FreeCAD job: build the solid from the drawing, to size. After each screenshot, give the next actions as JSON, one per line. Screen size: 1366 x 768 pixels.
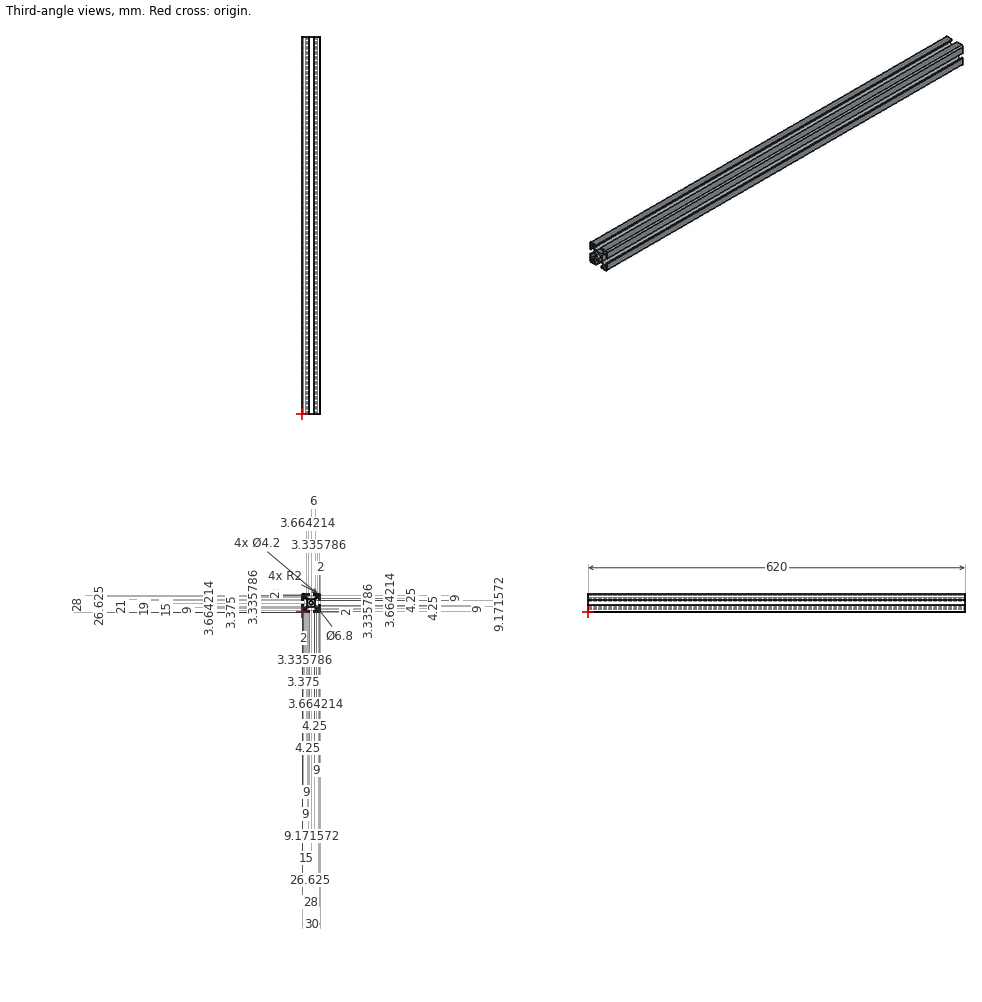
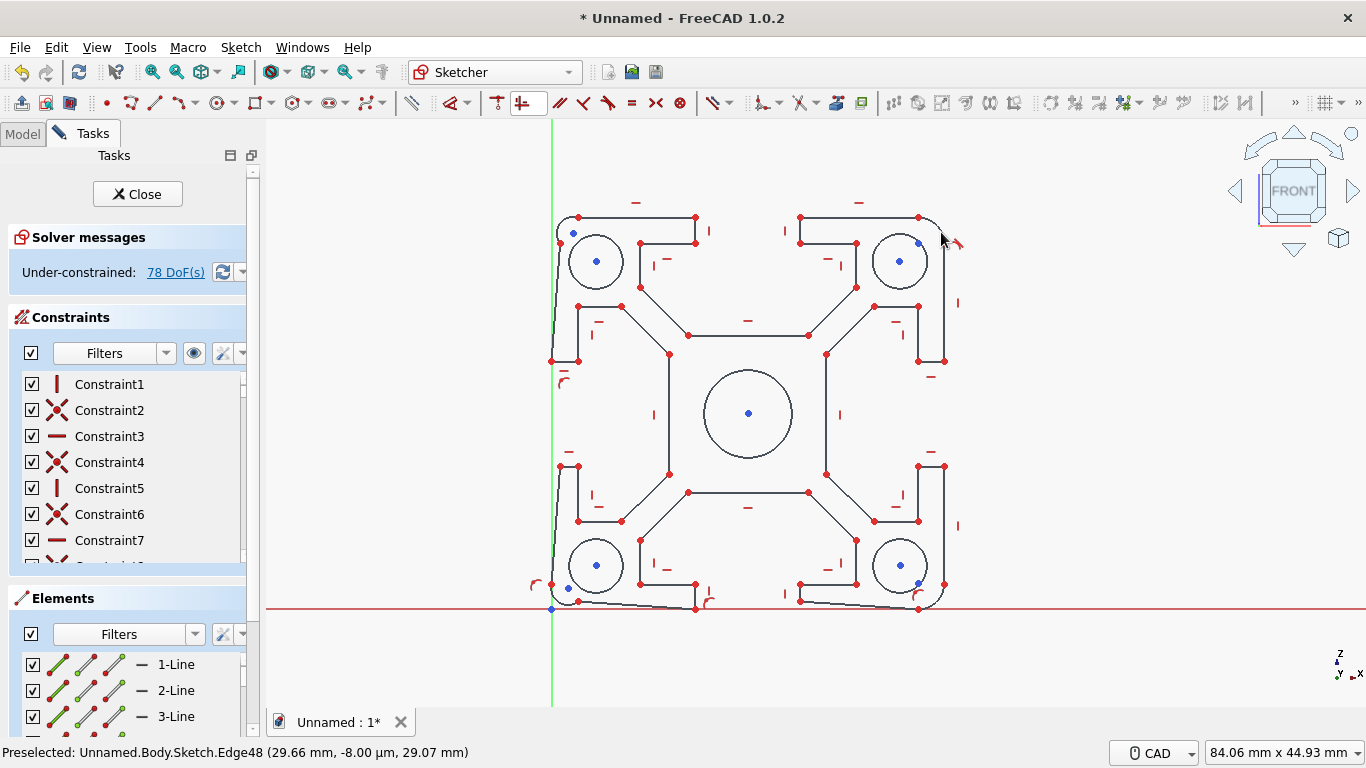
{"action": "left_click", "coordinate": [944, 502]}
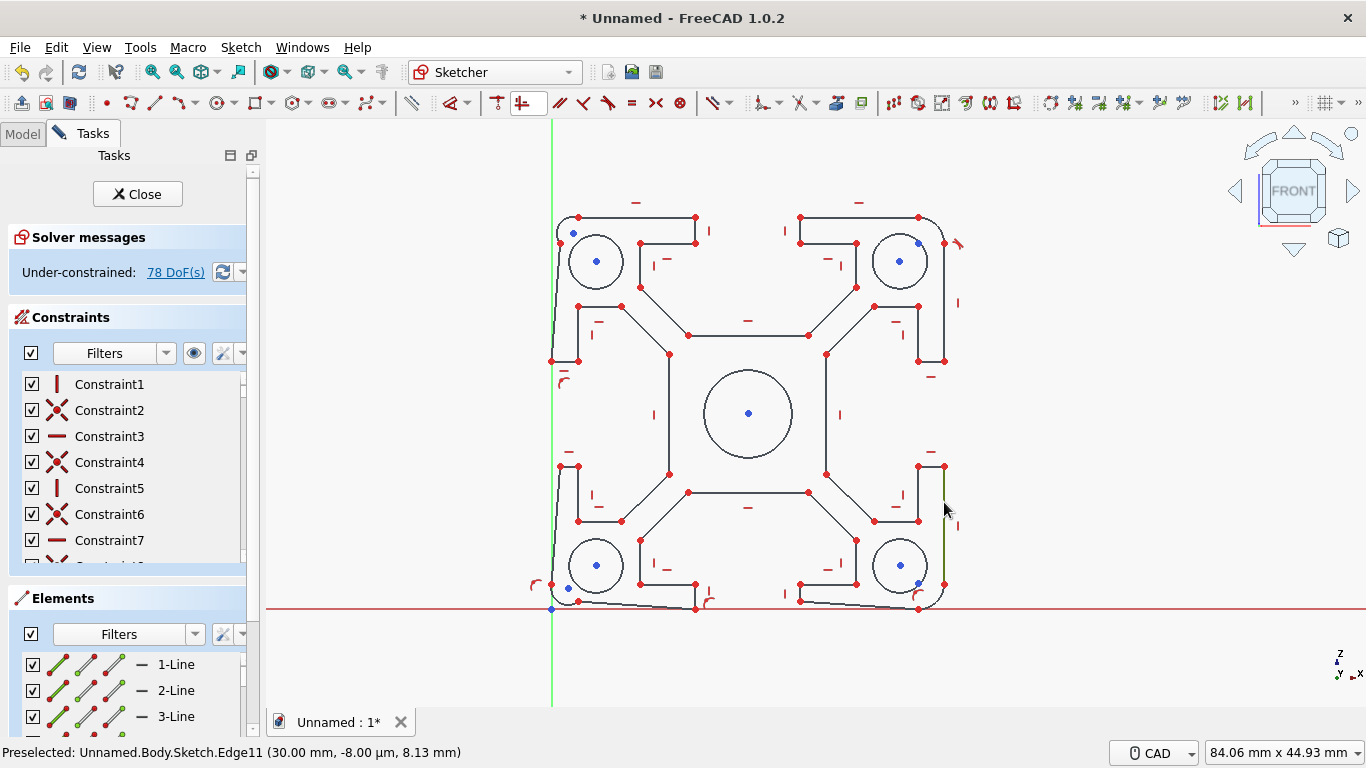
{"action": "left_click", "coordinate": [930, 607]}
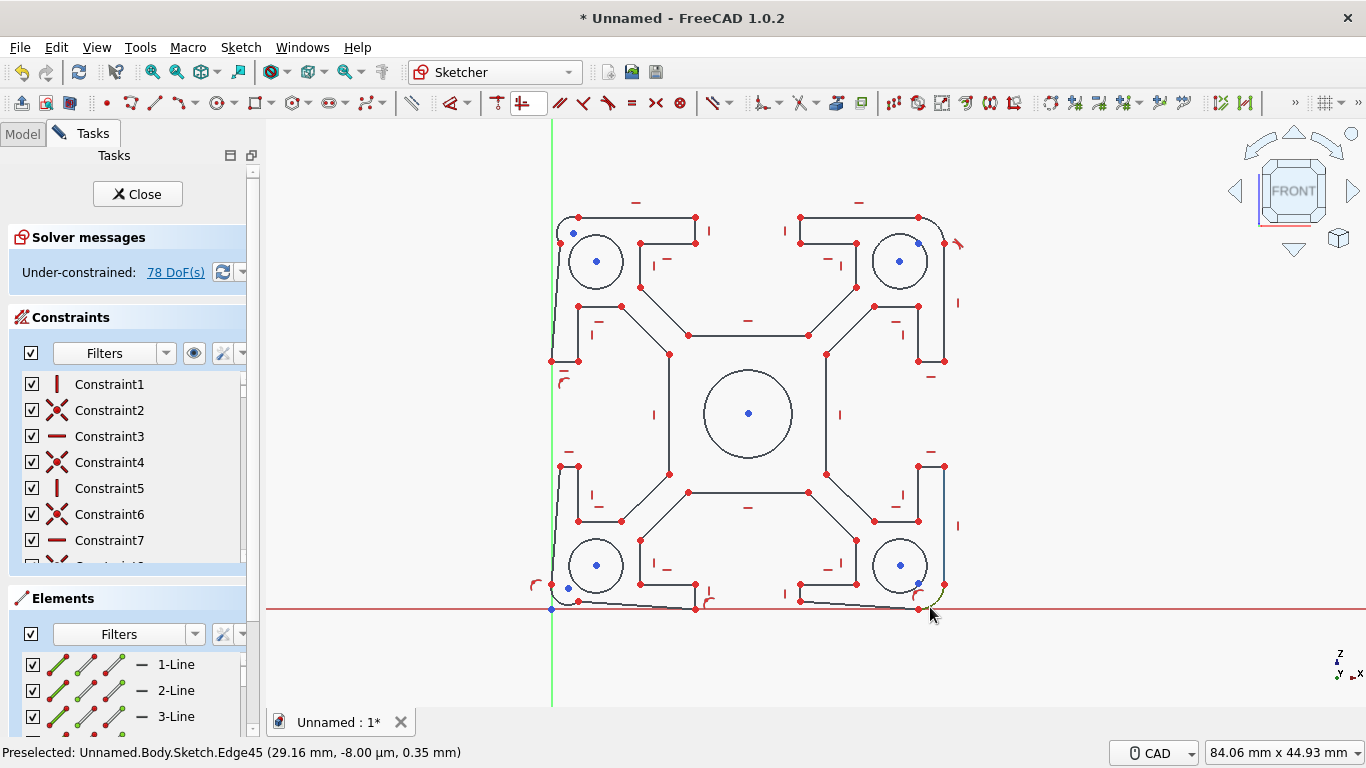
{"action": "key", "text": "t"}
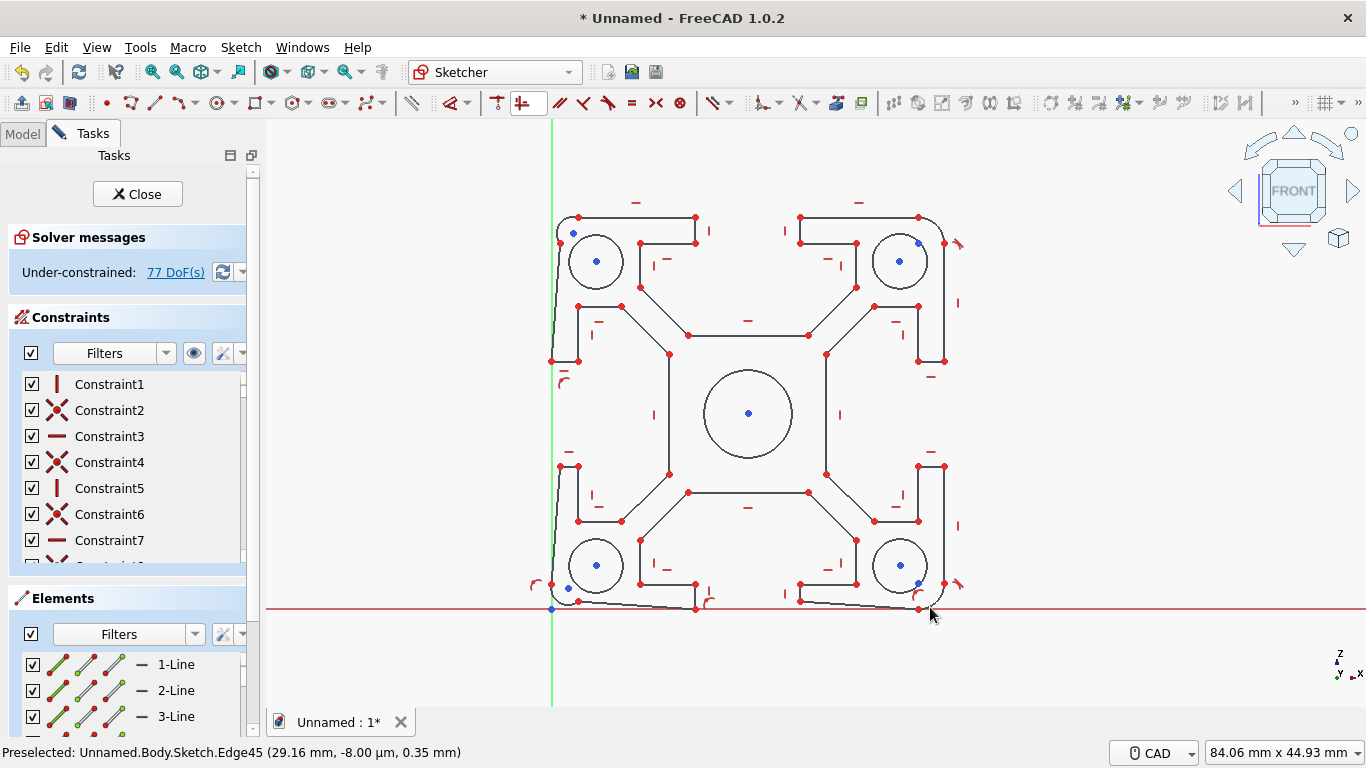
{"action": "left_click", "coordinate": [883, 607]}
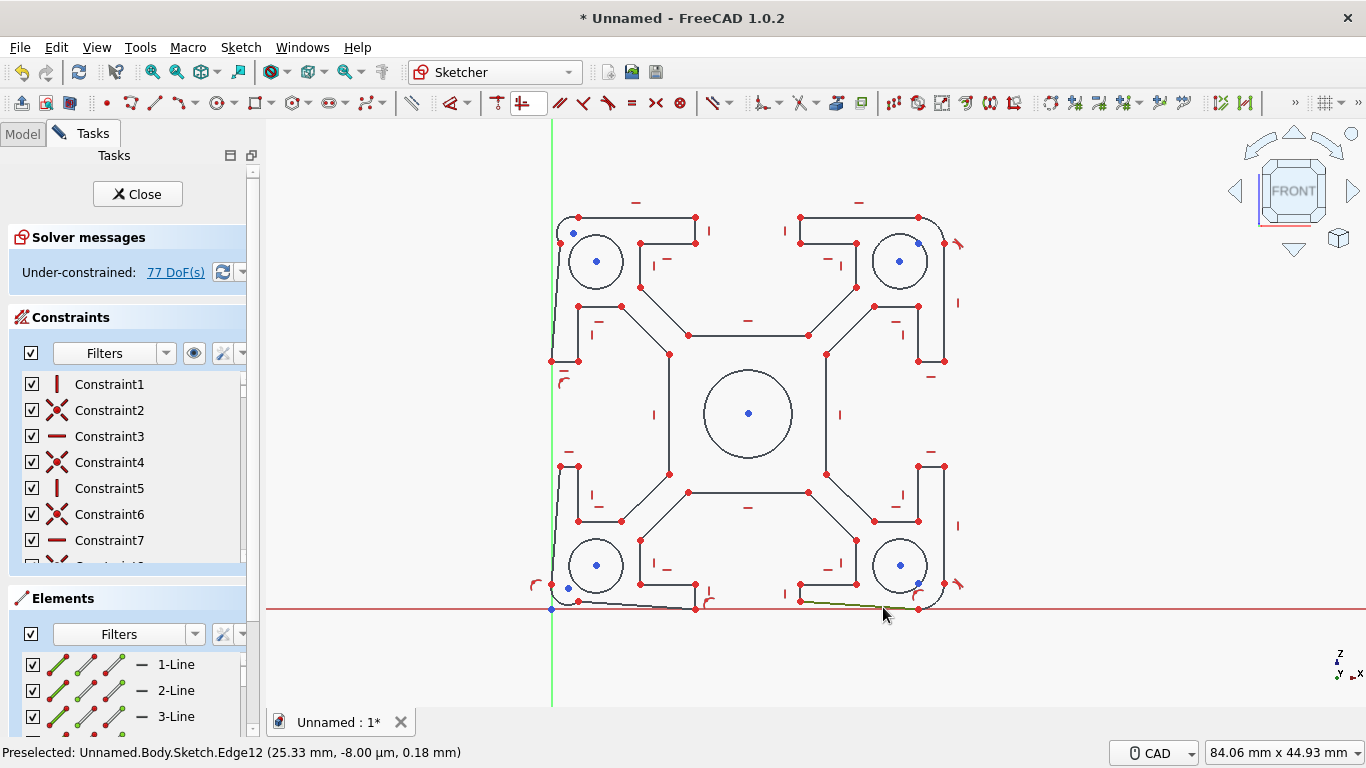
{"action": "left_click", "coordinate": [930, 607]}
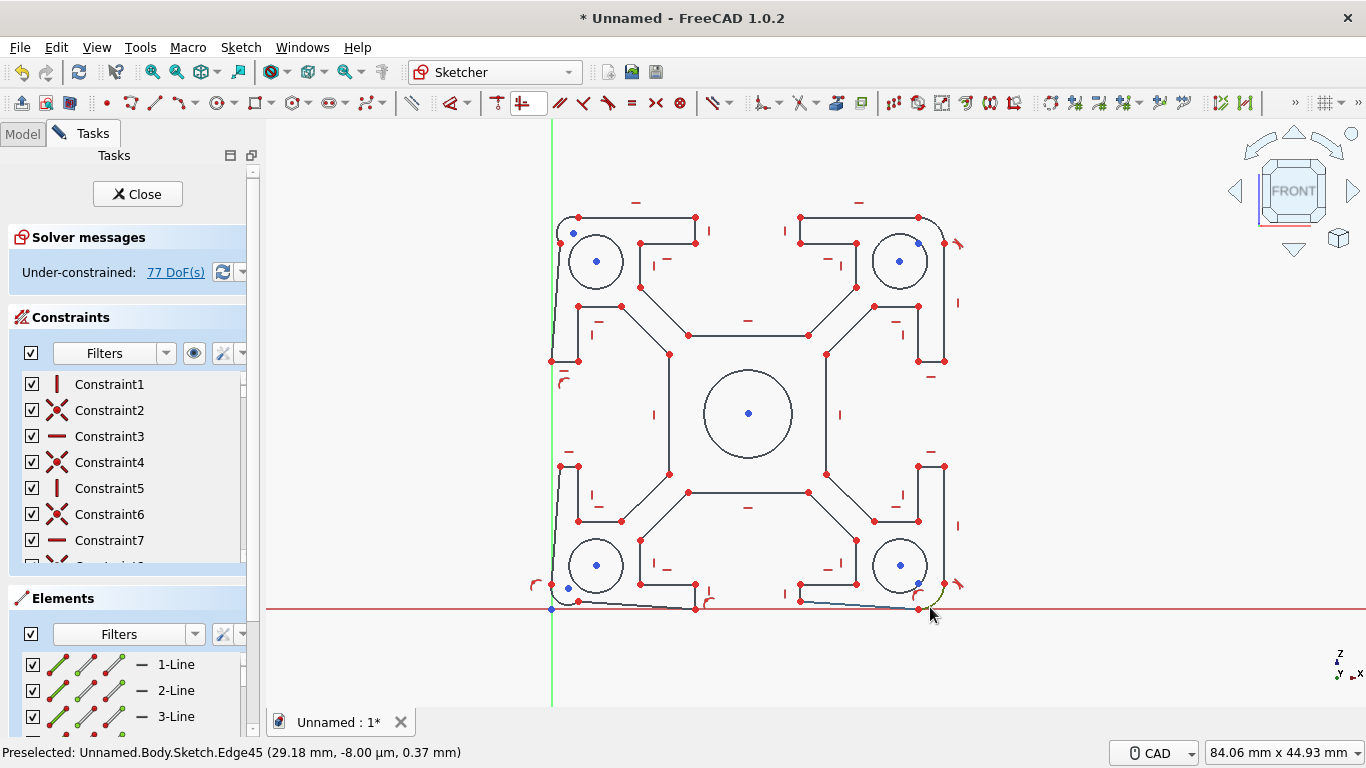
{"action": "key", "text": "t"}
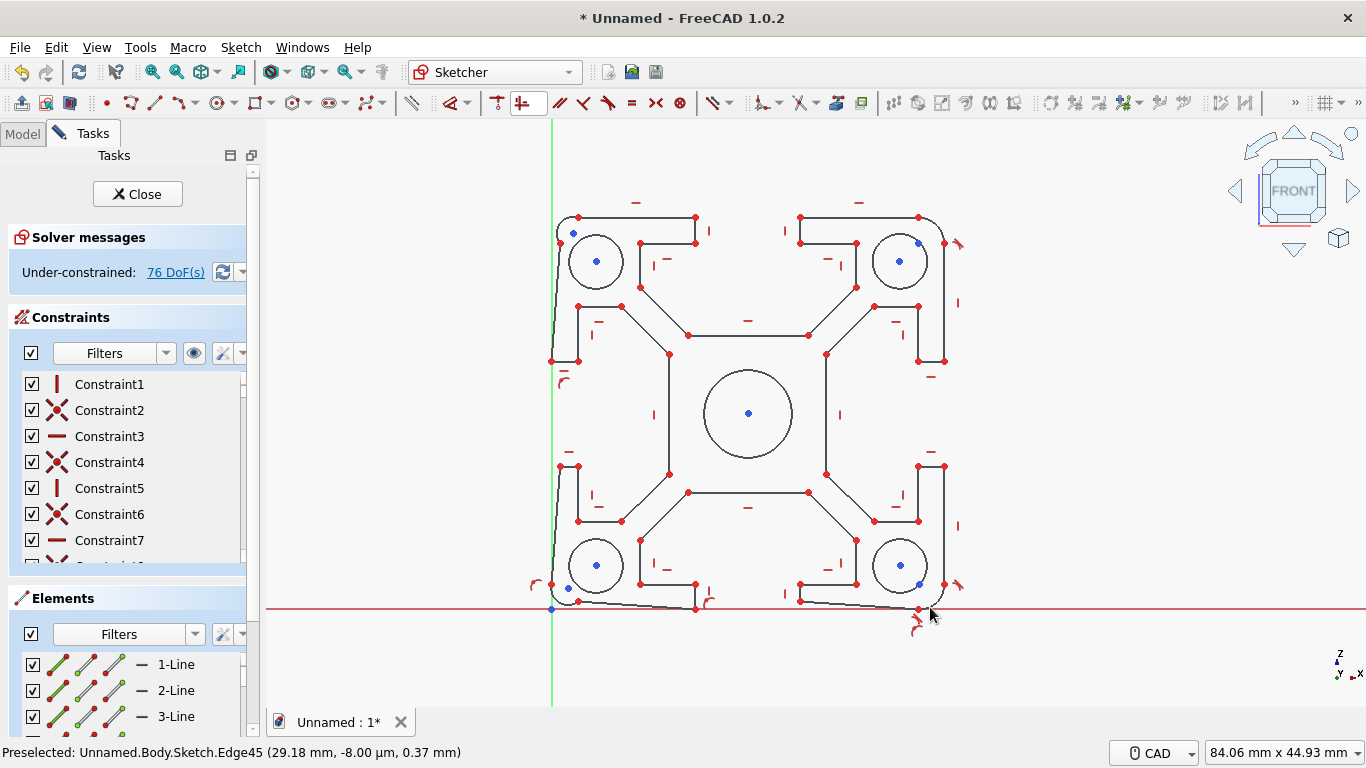
{"action": "left_click", "coordinate": [660, 607]}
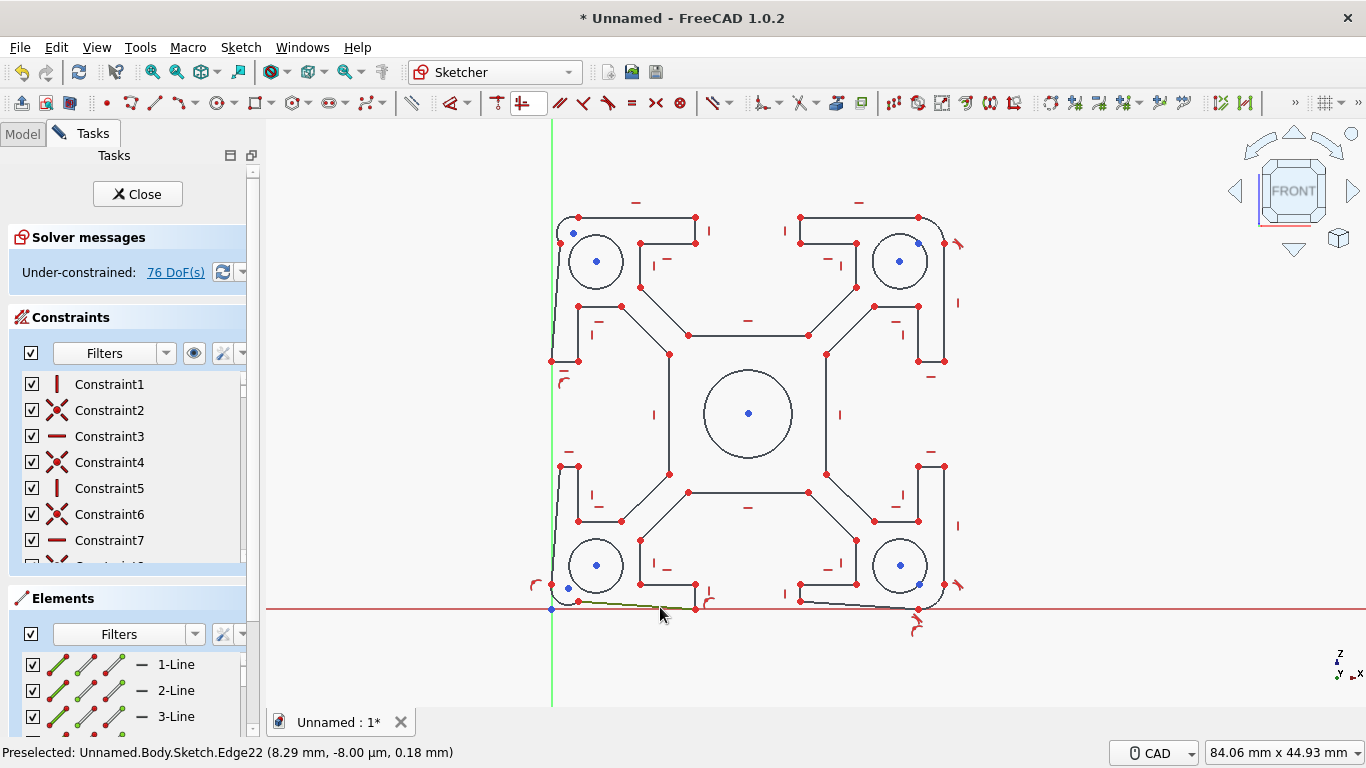
{"action": "left_click", "coordinate": [553, 596]}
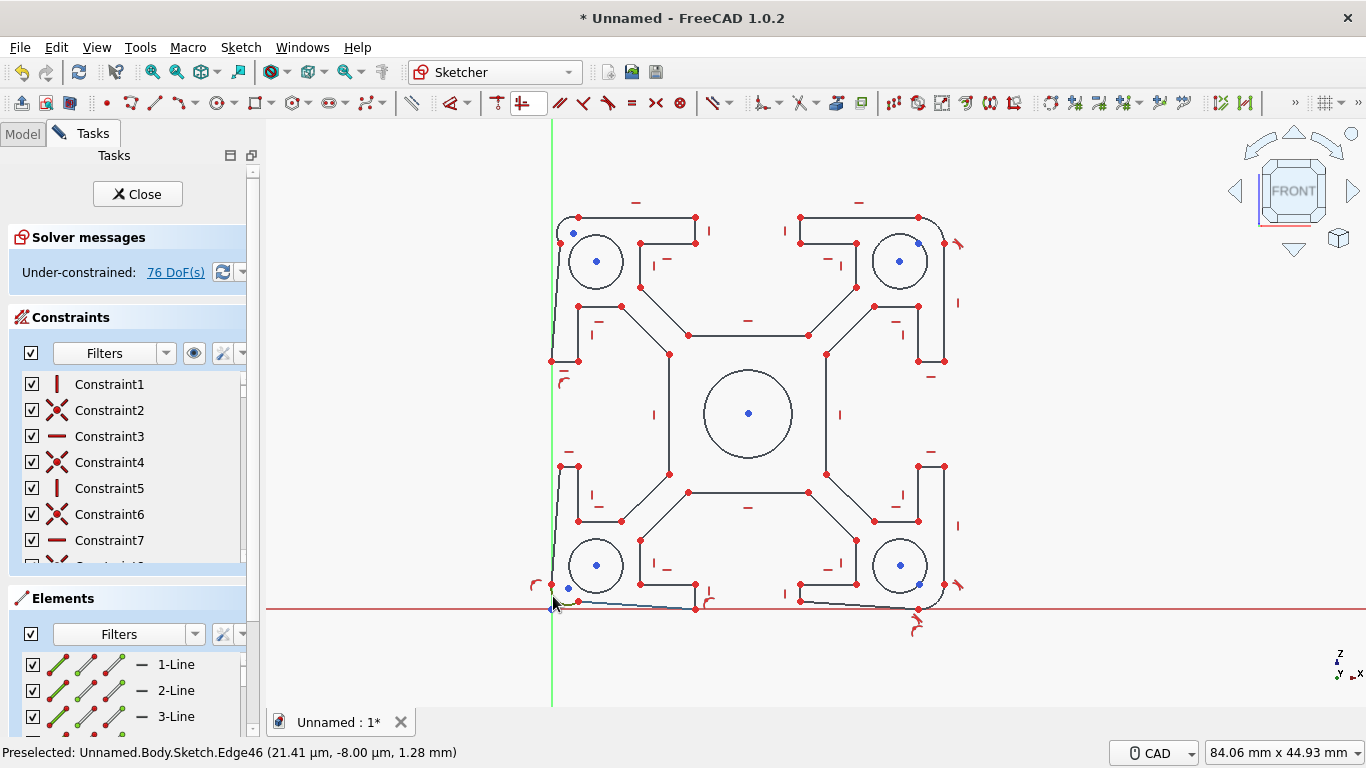
{"action": "key", "text": "t"}